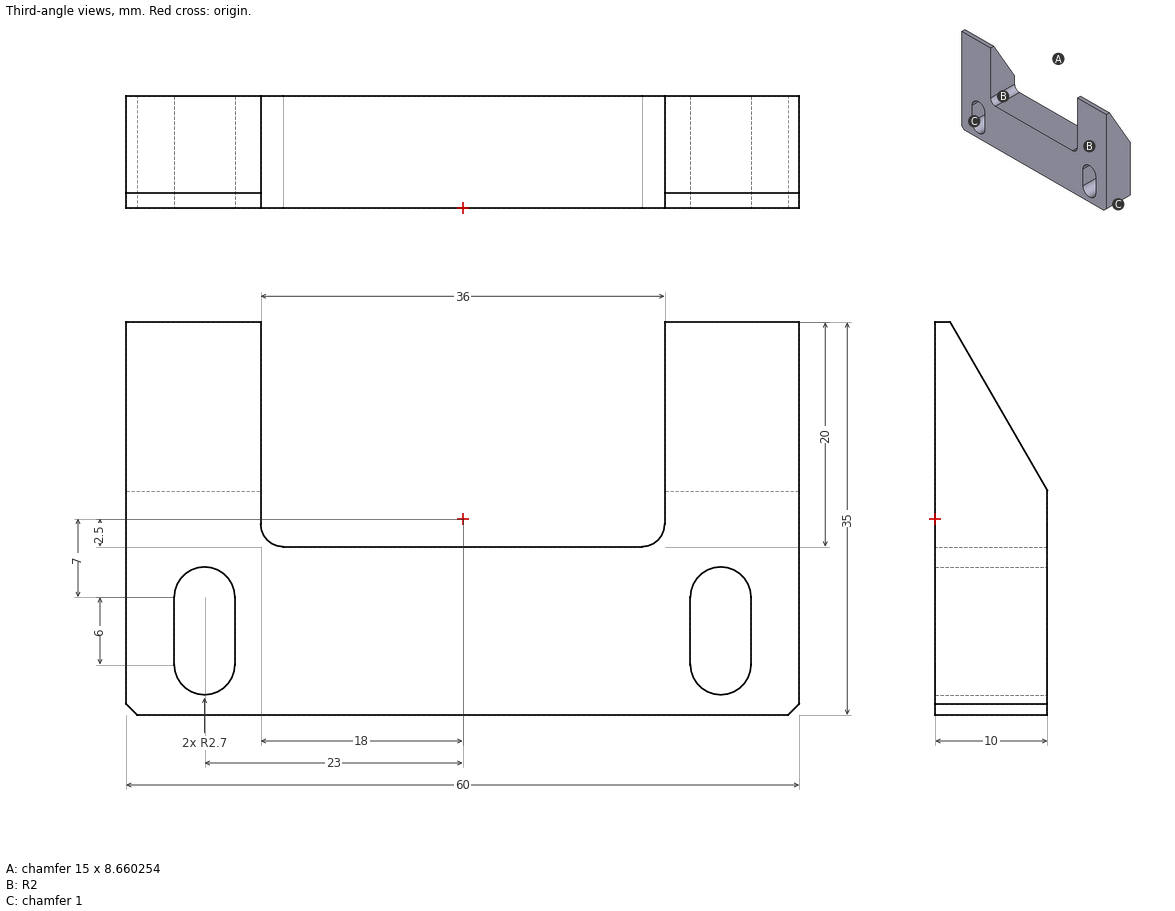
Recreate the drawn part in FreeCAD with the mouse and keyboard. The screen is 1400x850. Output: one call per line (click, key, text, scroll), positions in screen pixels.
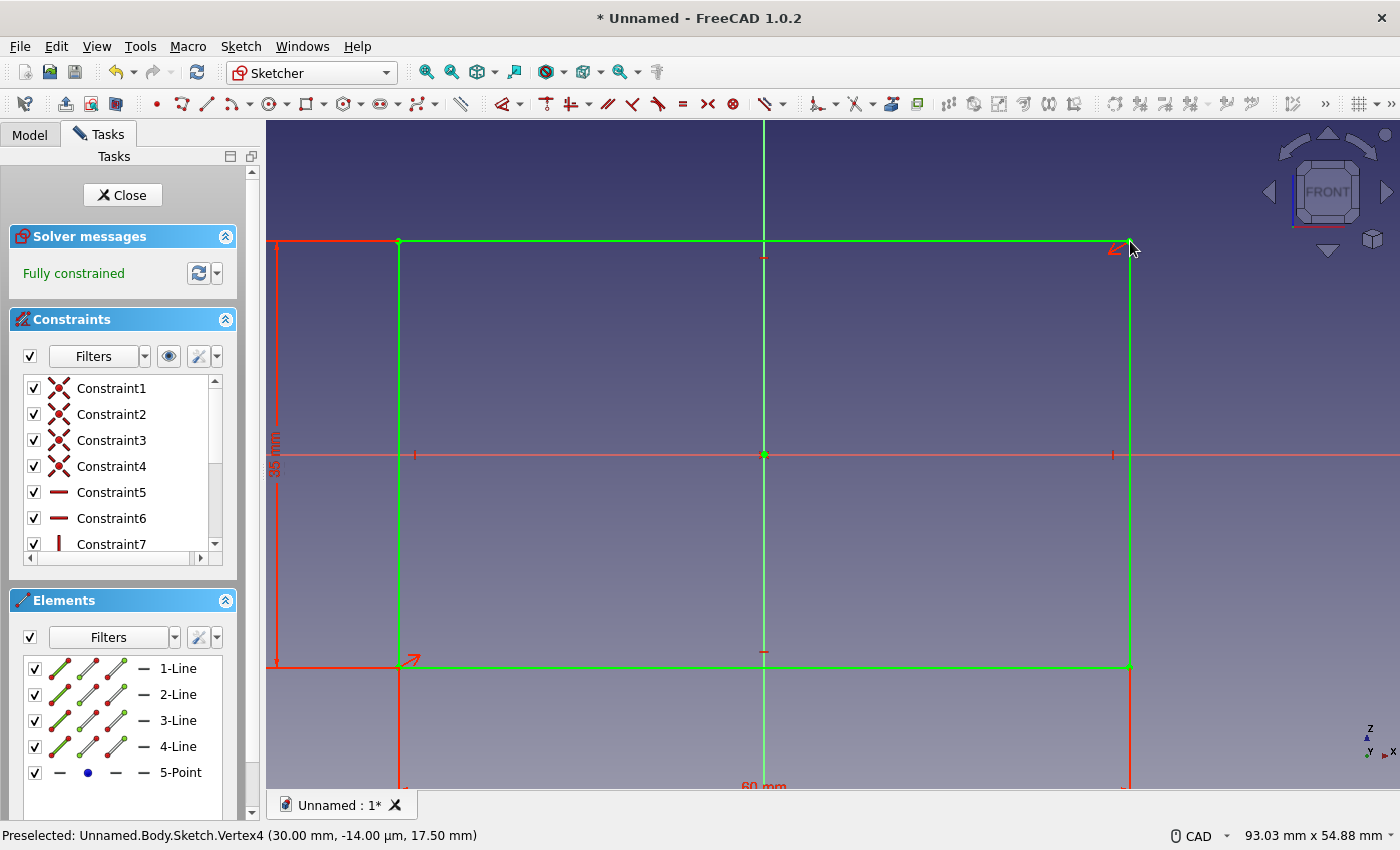
click(123, 195)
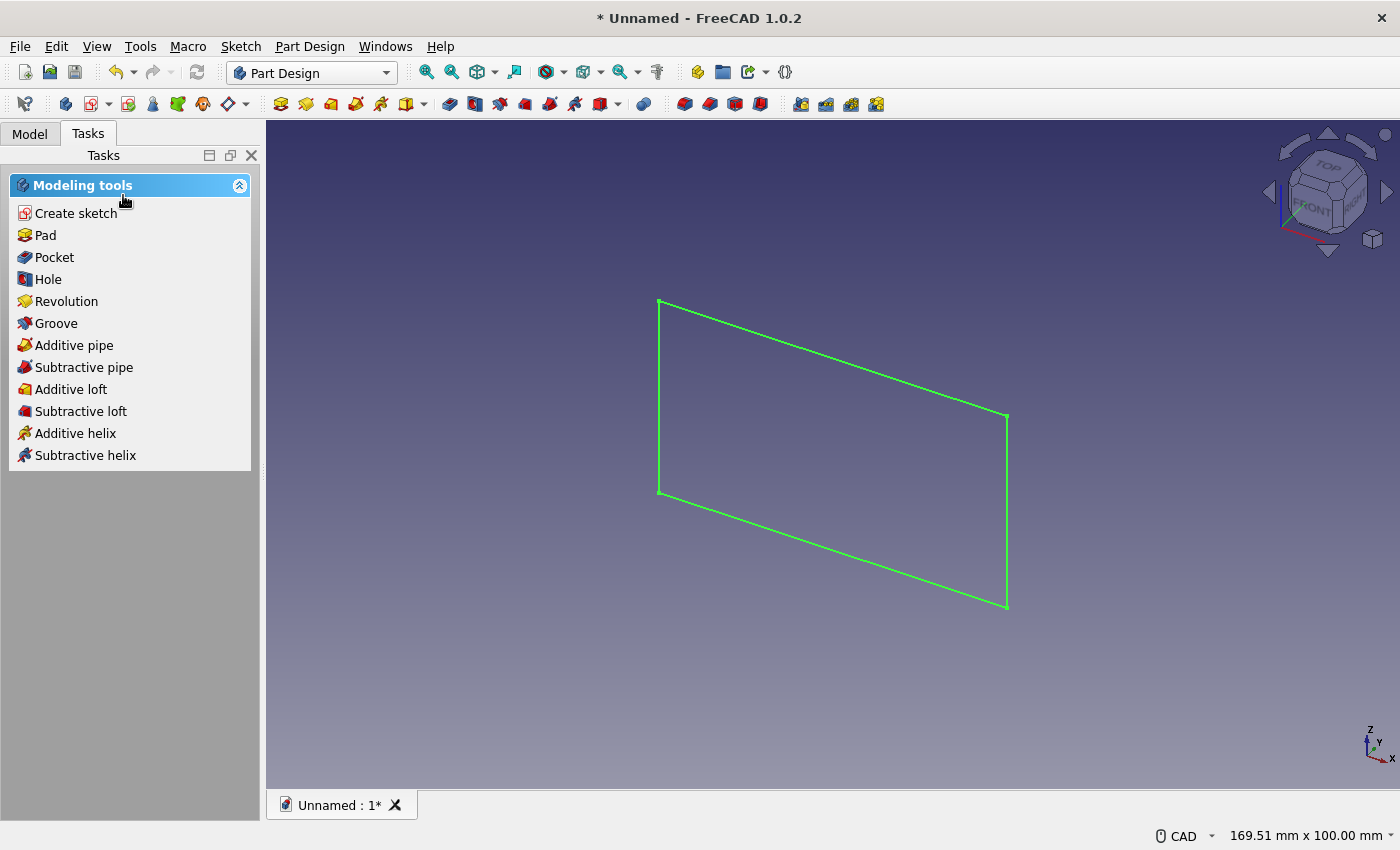
click(281, 104)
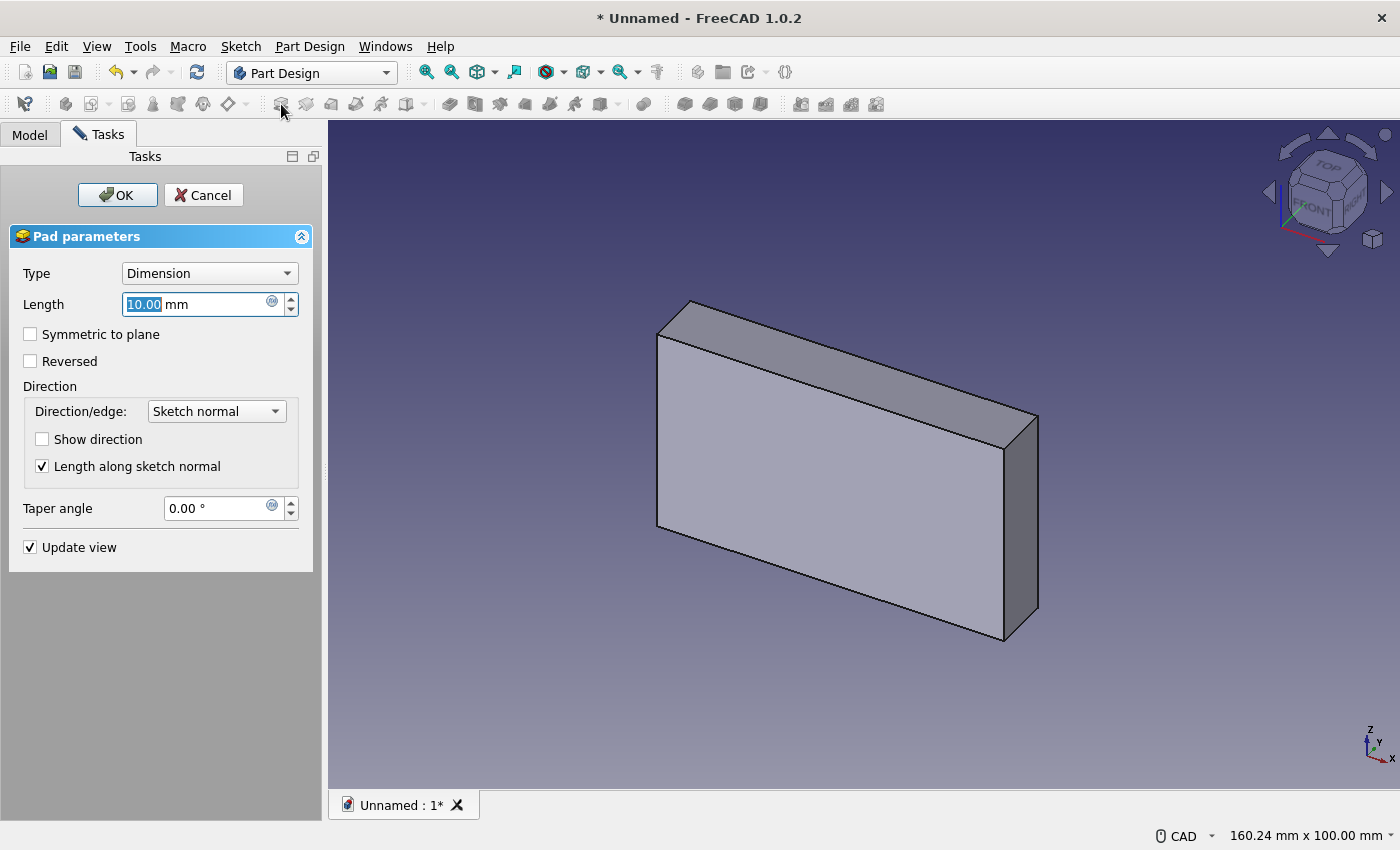
text(10)
key(Tab)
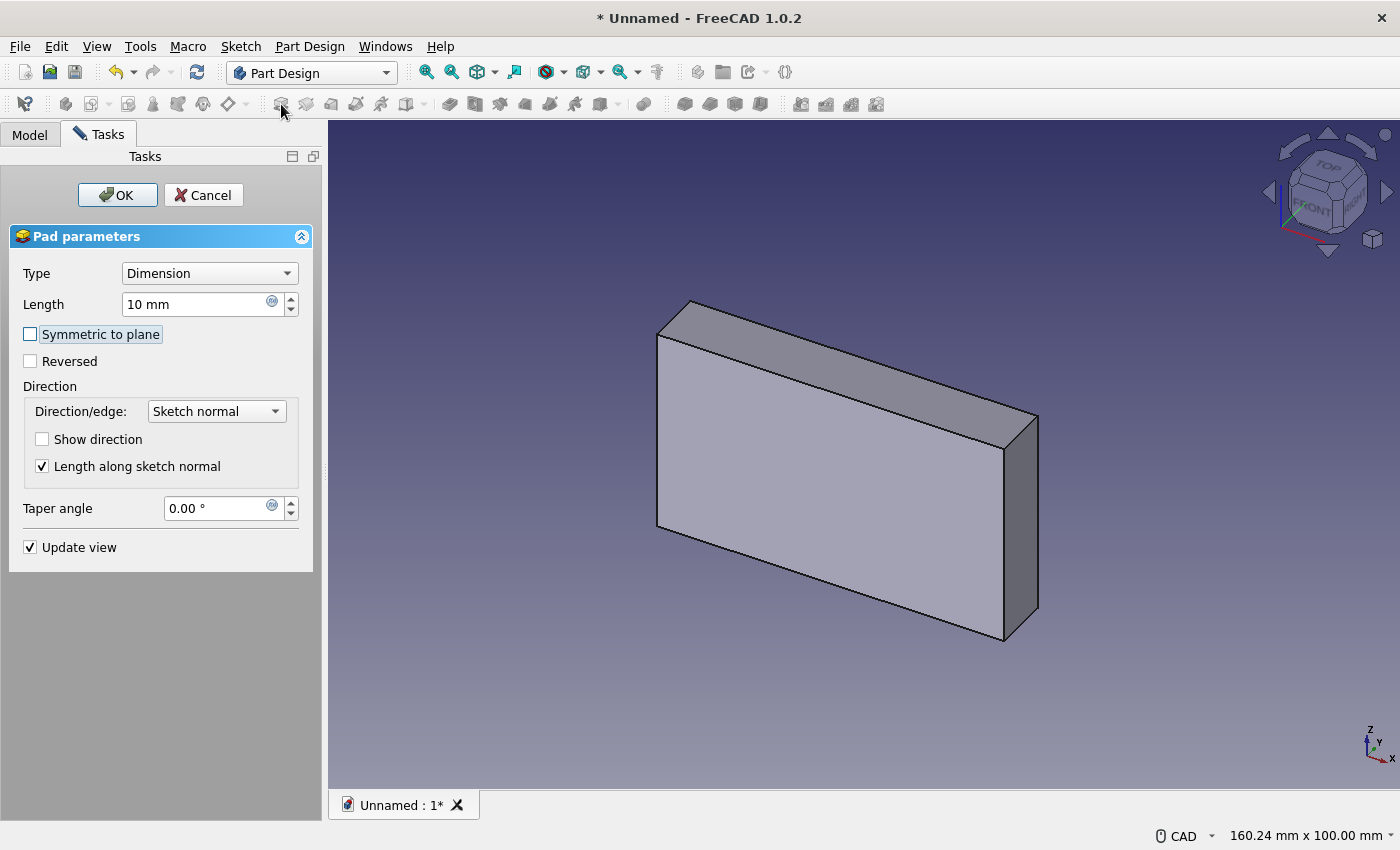
click(31, 361)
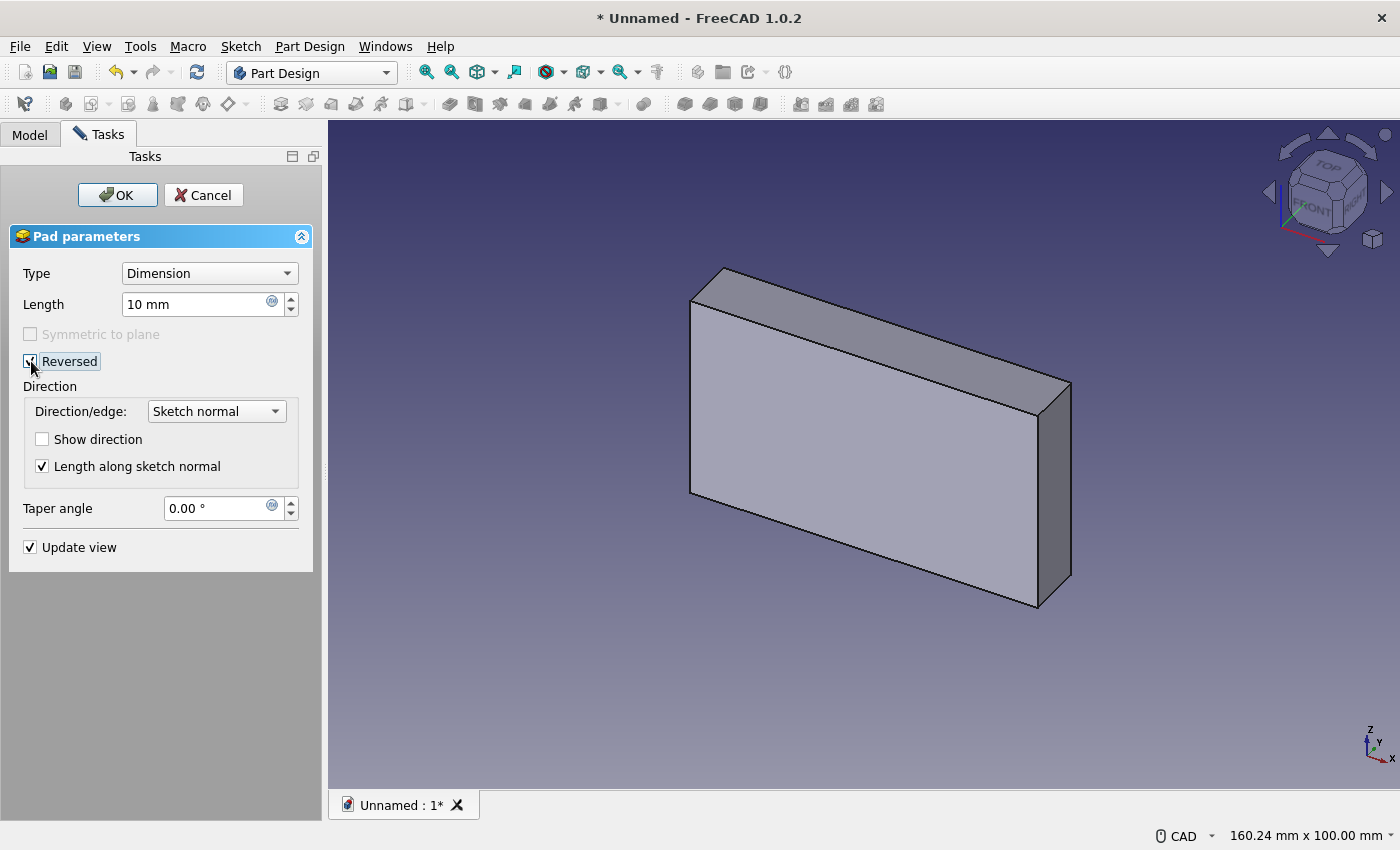
click(118, 195)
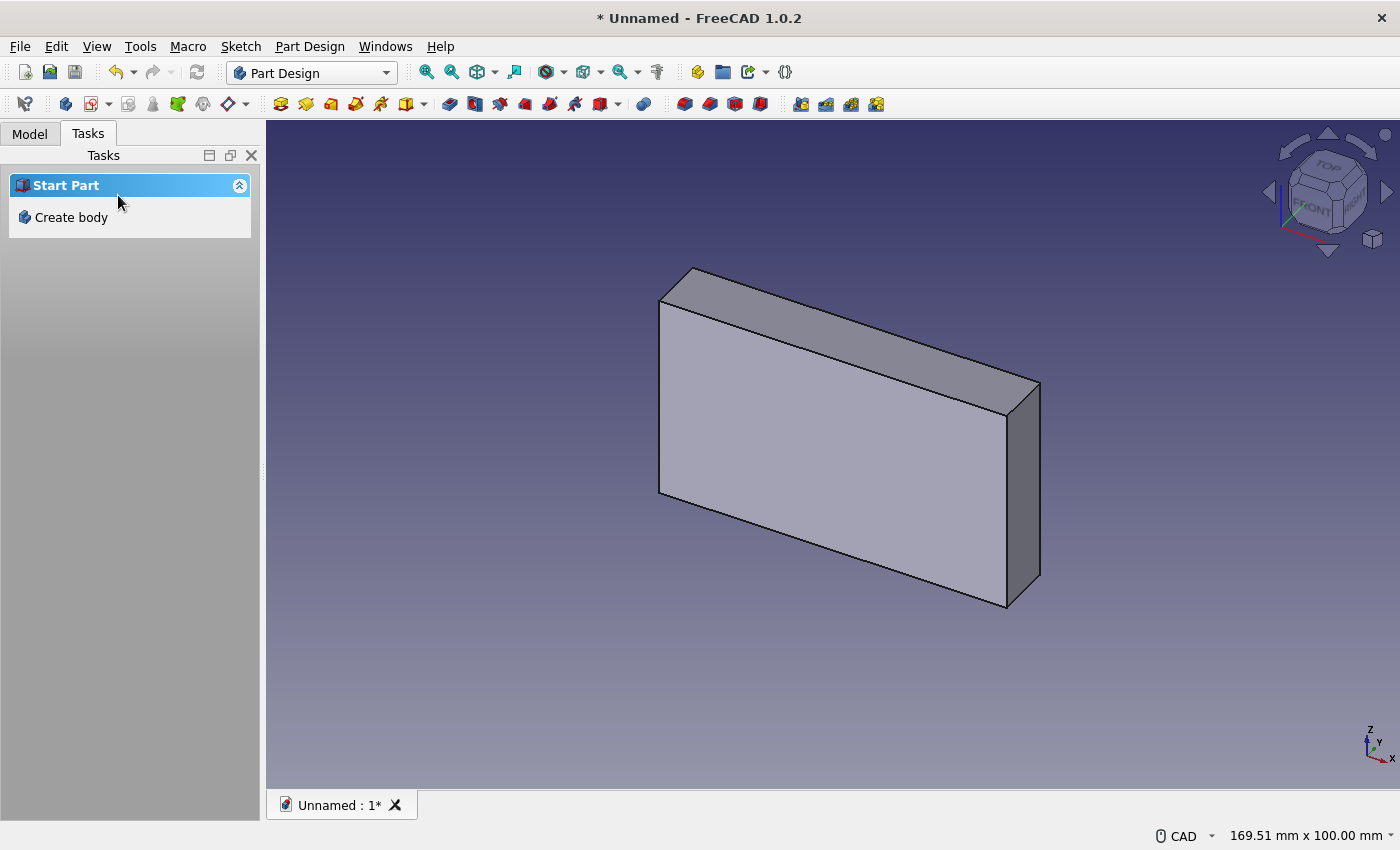
key(0)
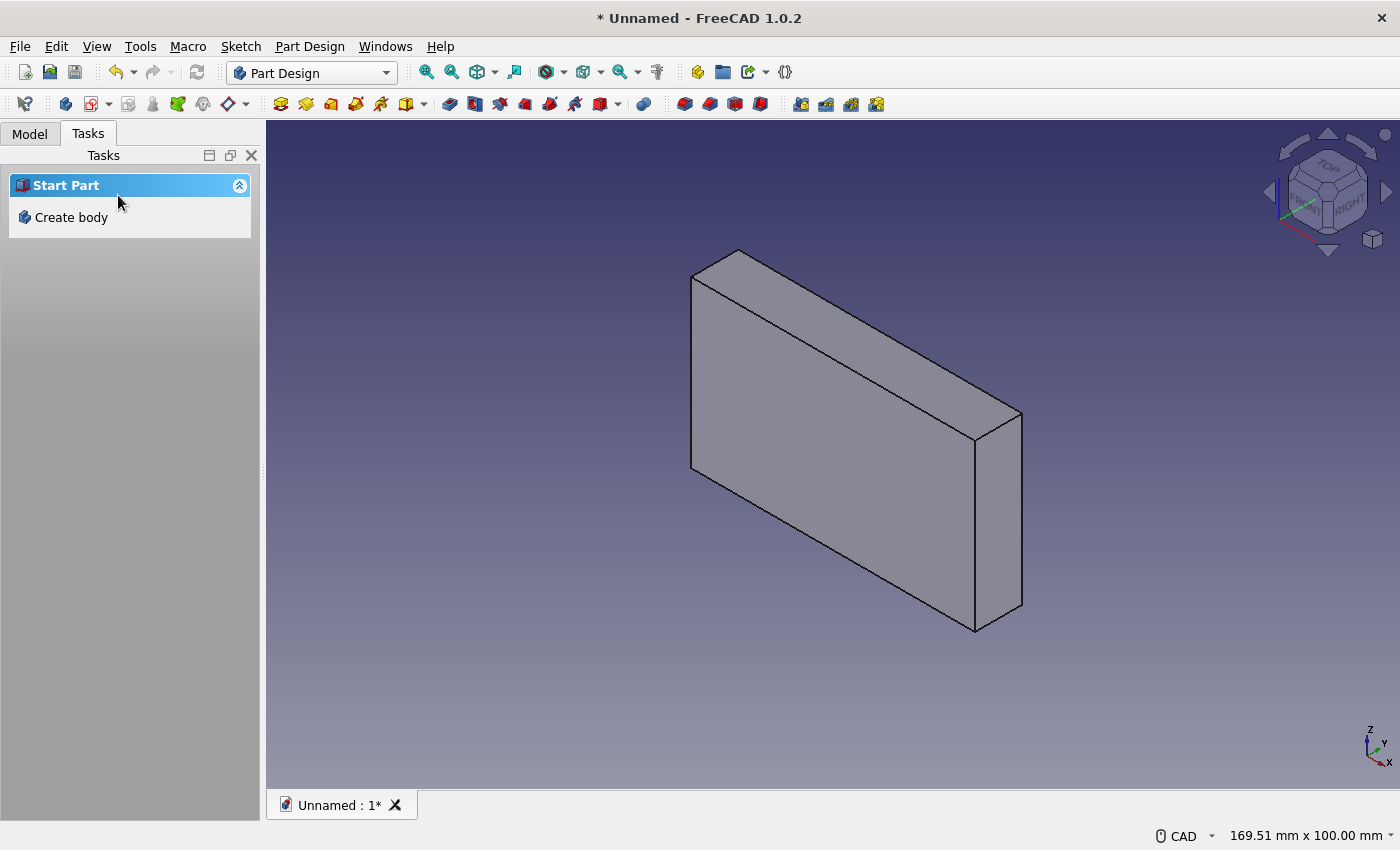
key(2)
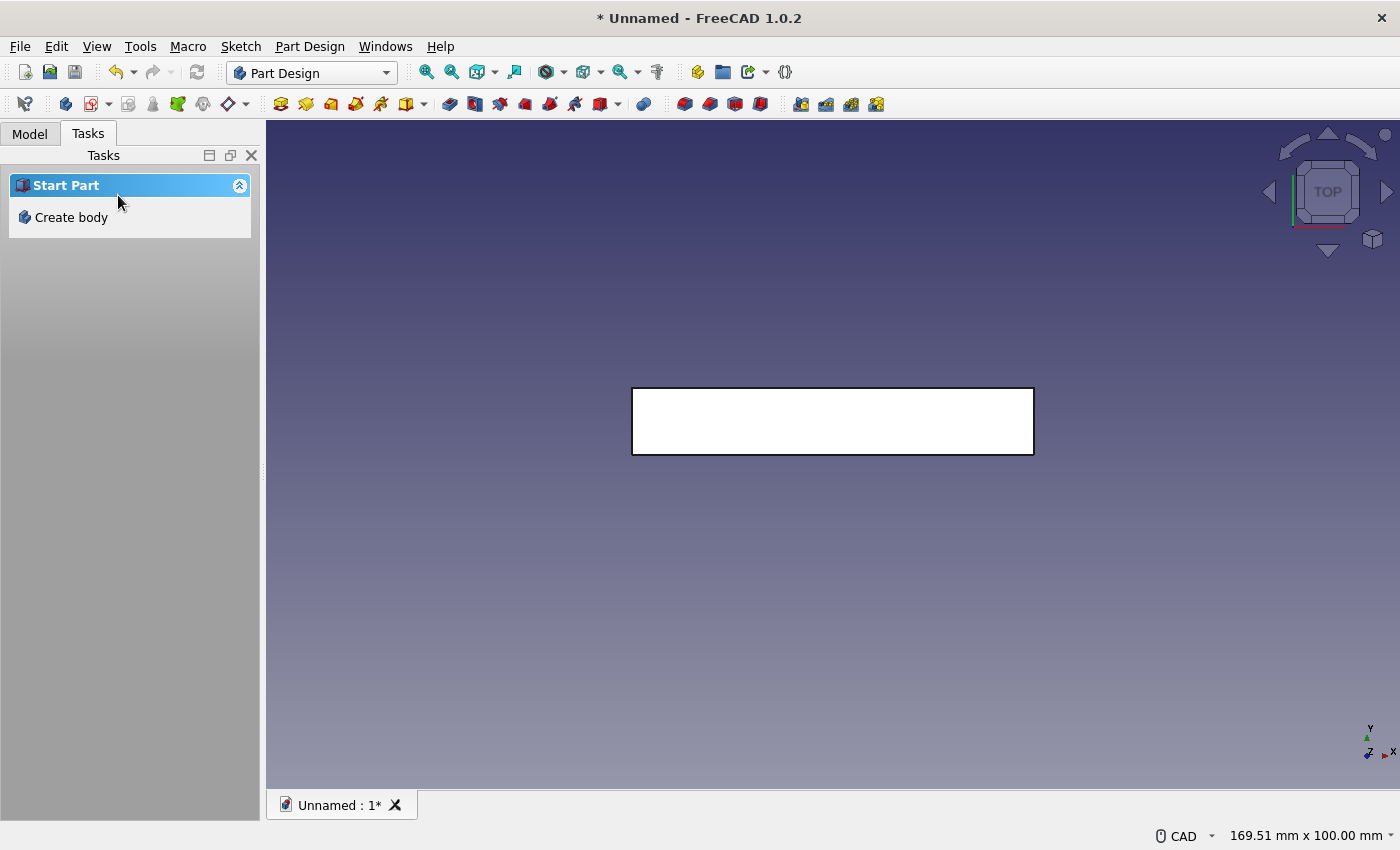
click(427, 72)